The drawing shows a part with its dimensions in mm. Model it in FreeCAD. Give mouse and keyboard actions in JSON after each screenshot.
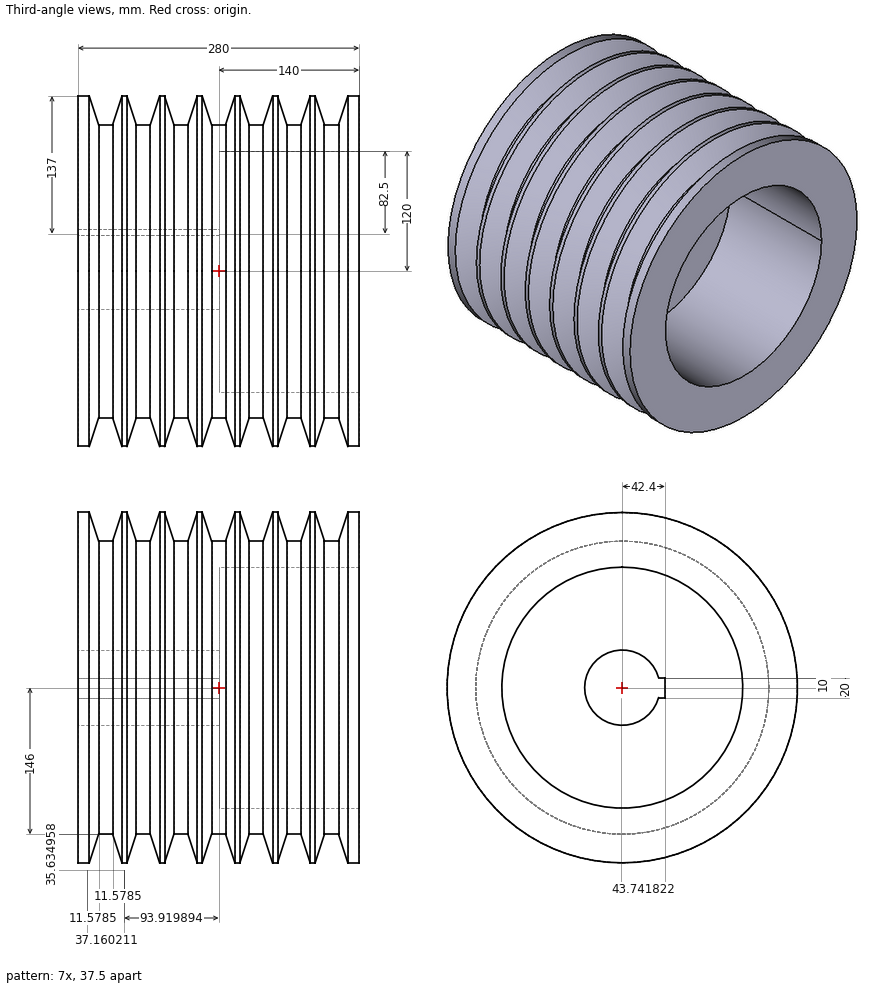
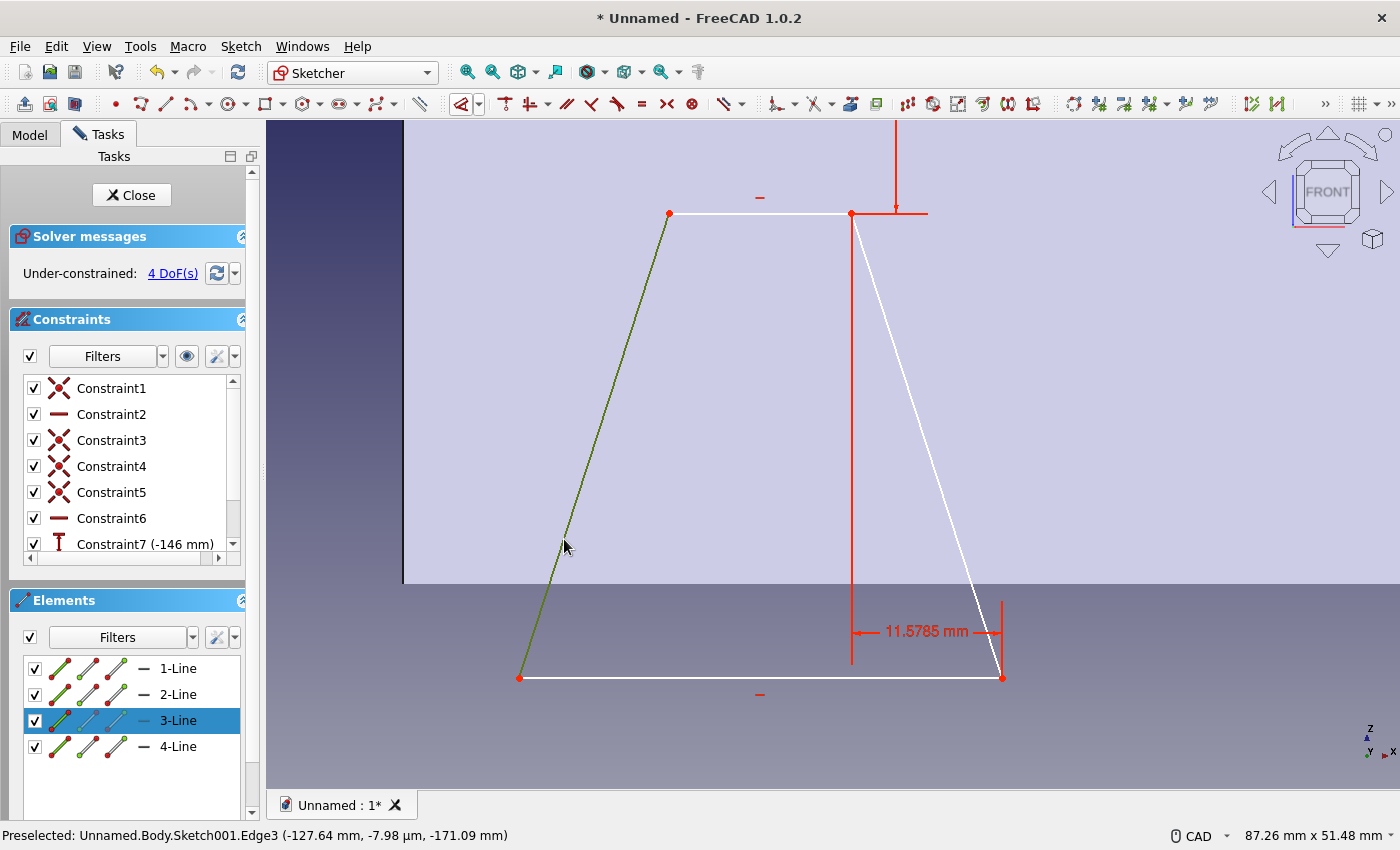
{"action": "left_click", "coordinate": [478, 104]}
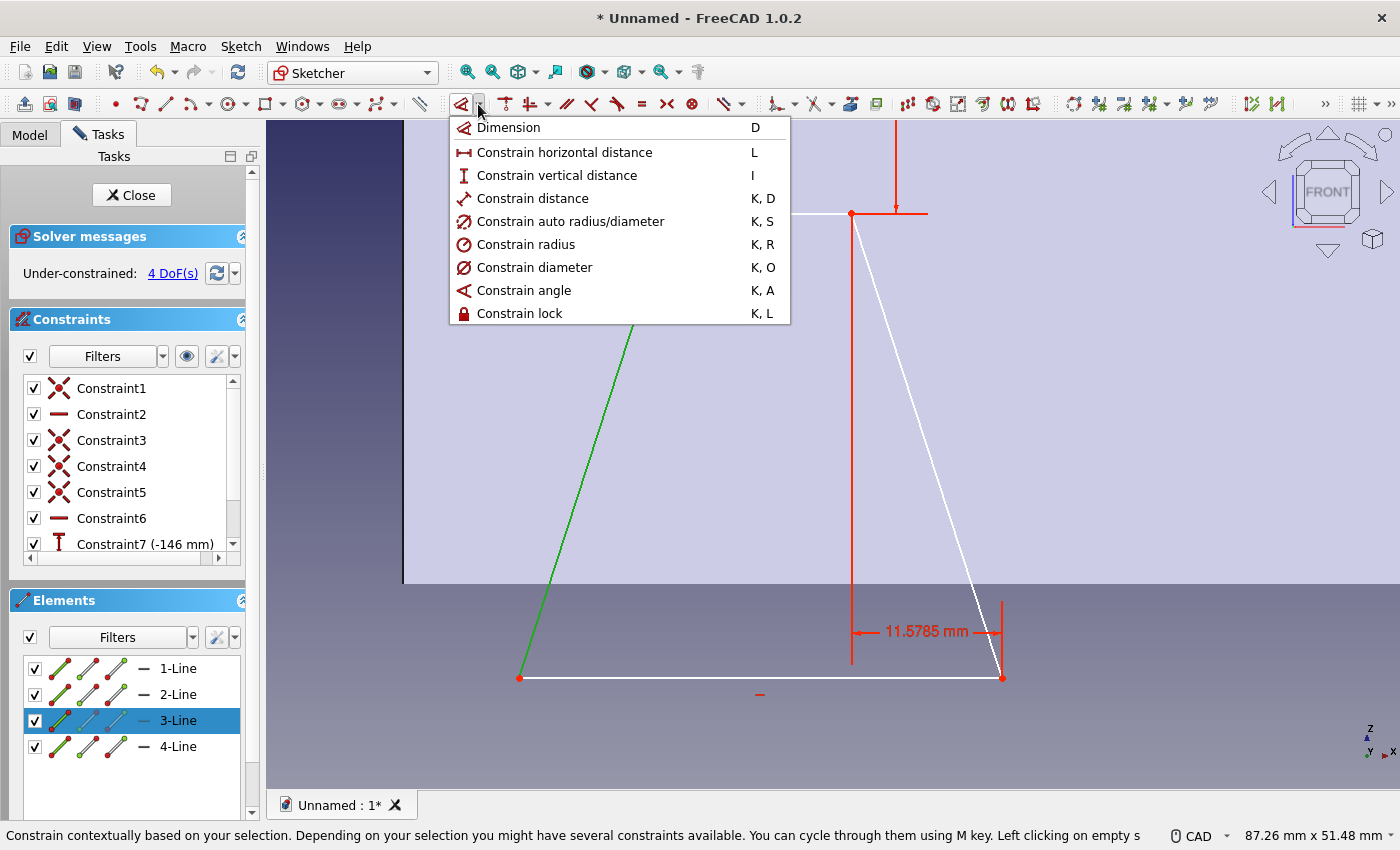
{"action": "left_click", "coordinate": [620, 152]}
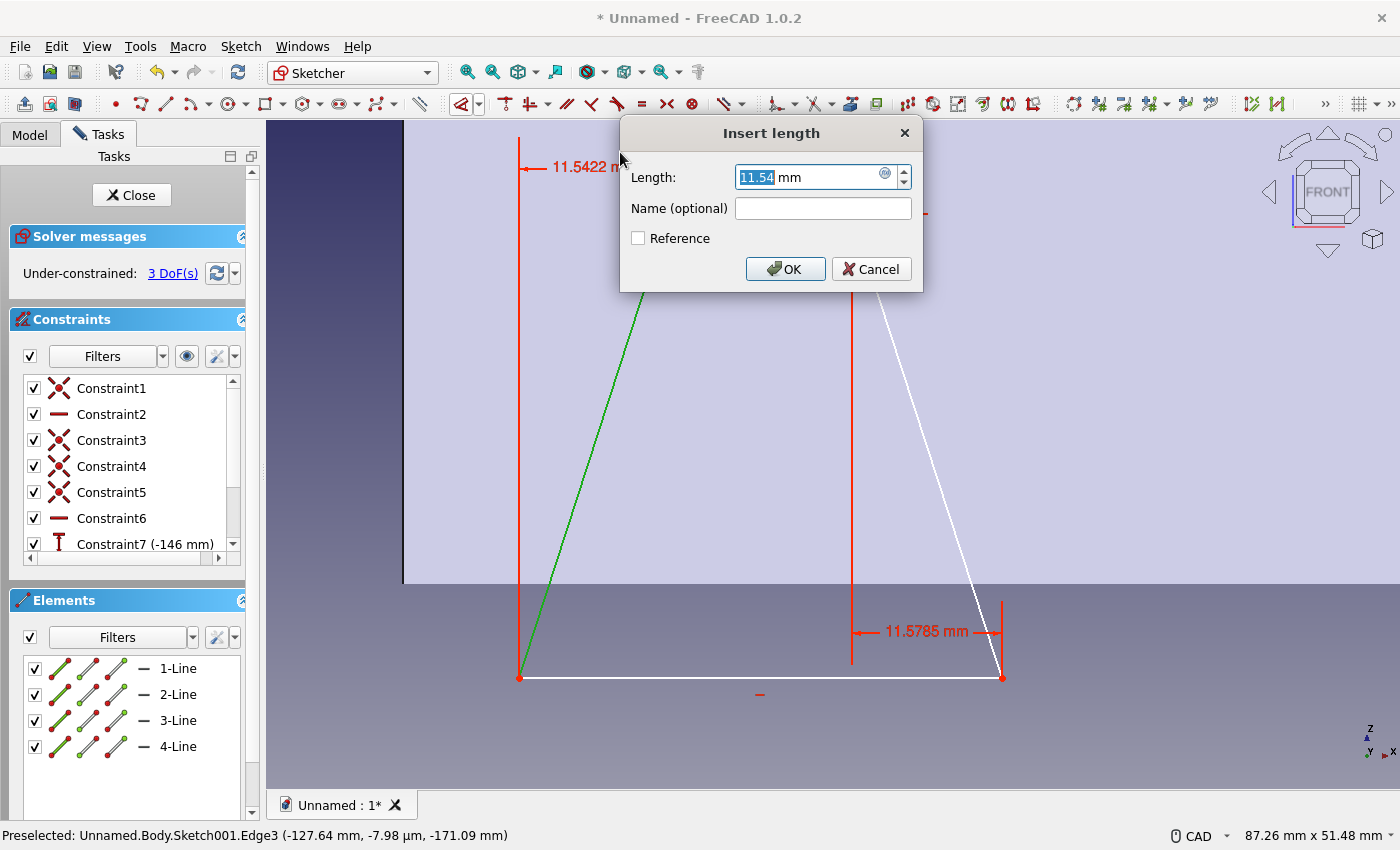
{"action": "type", "text": "11.5785"}
{"action": "key", "text": "Return"}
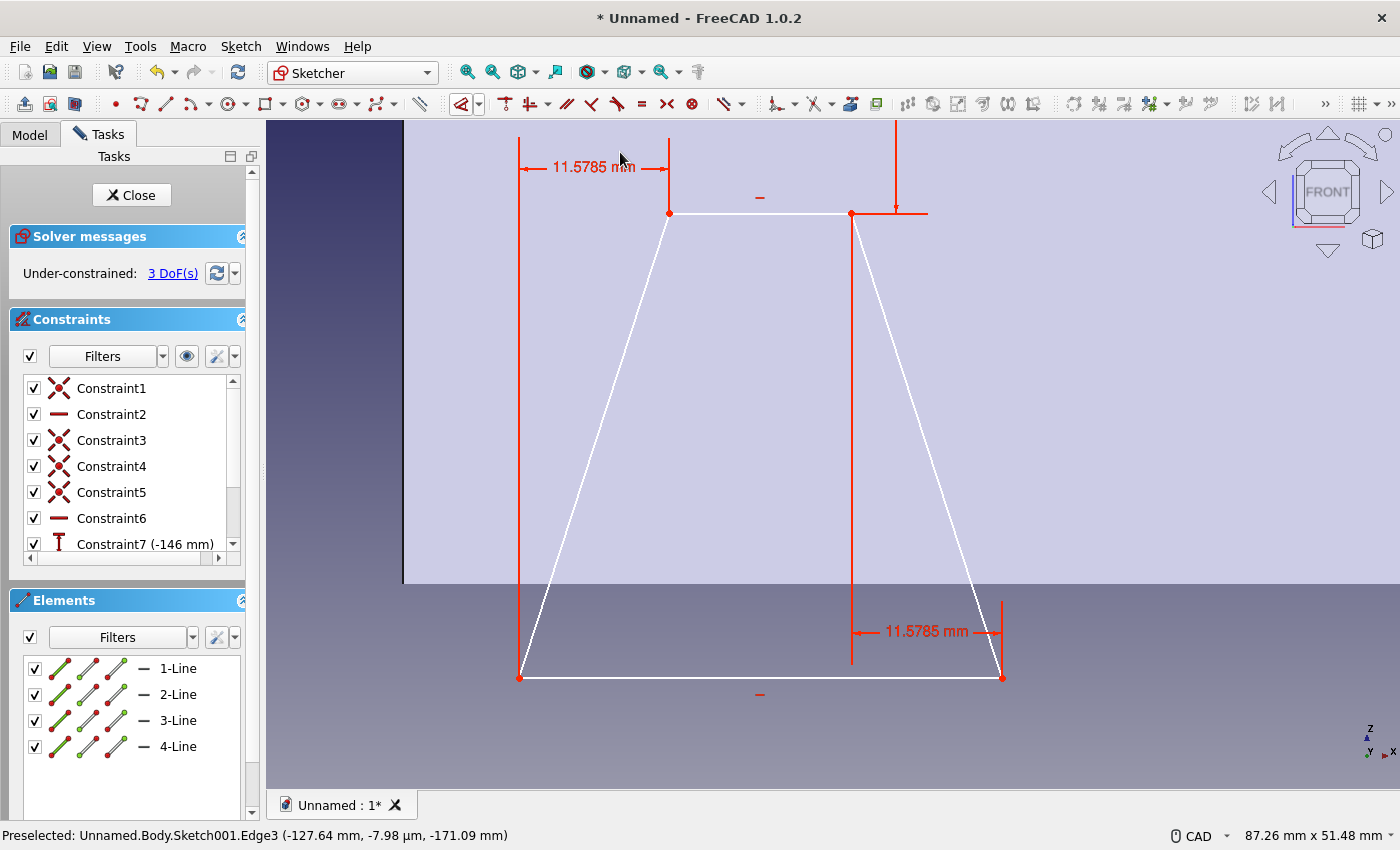
{"action": "left_click", "coordinate": [857, 678]}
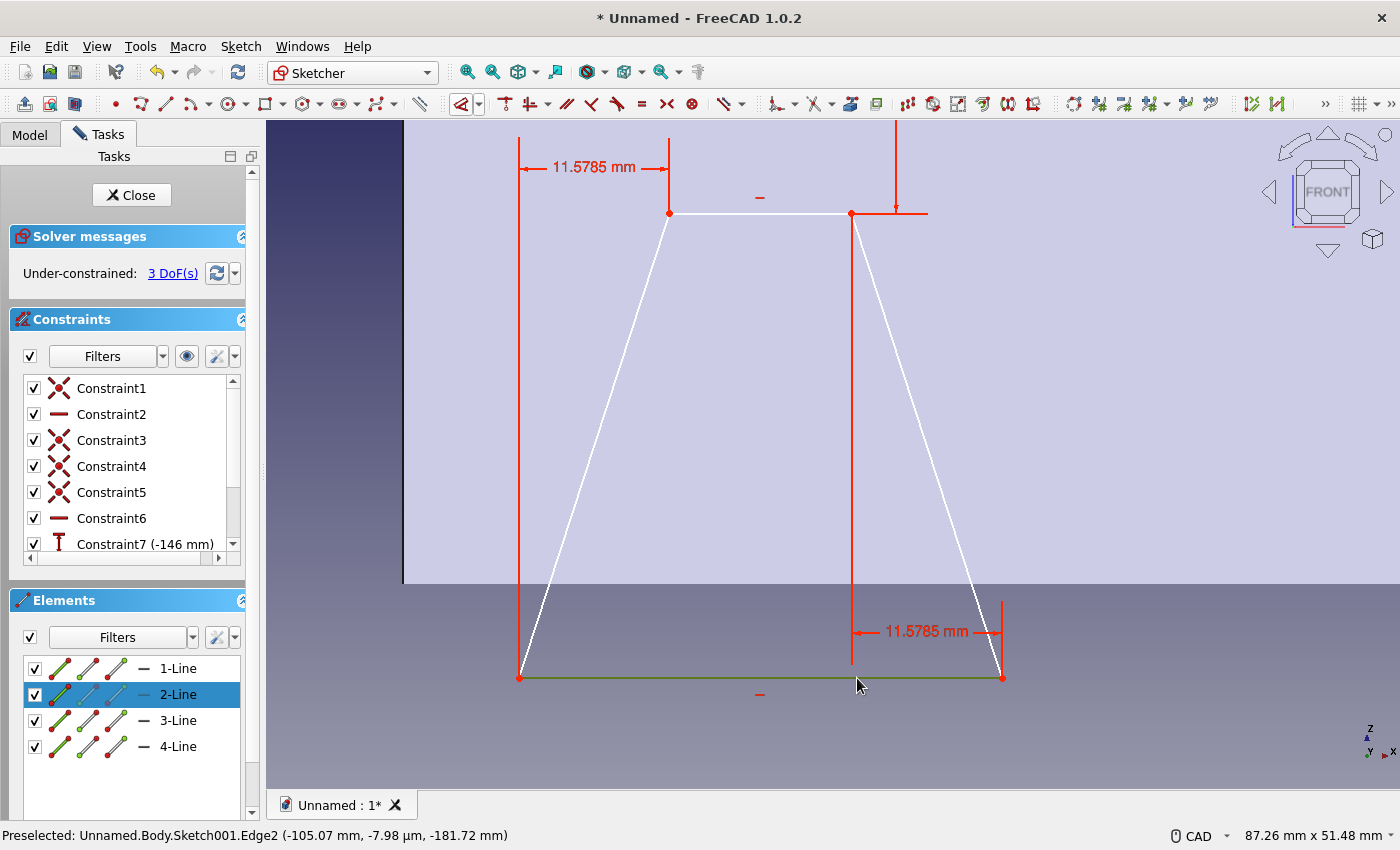
{"action": "left_click", "coordinate": [478, 104]}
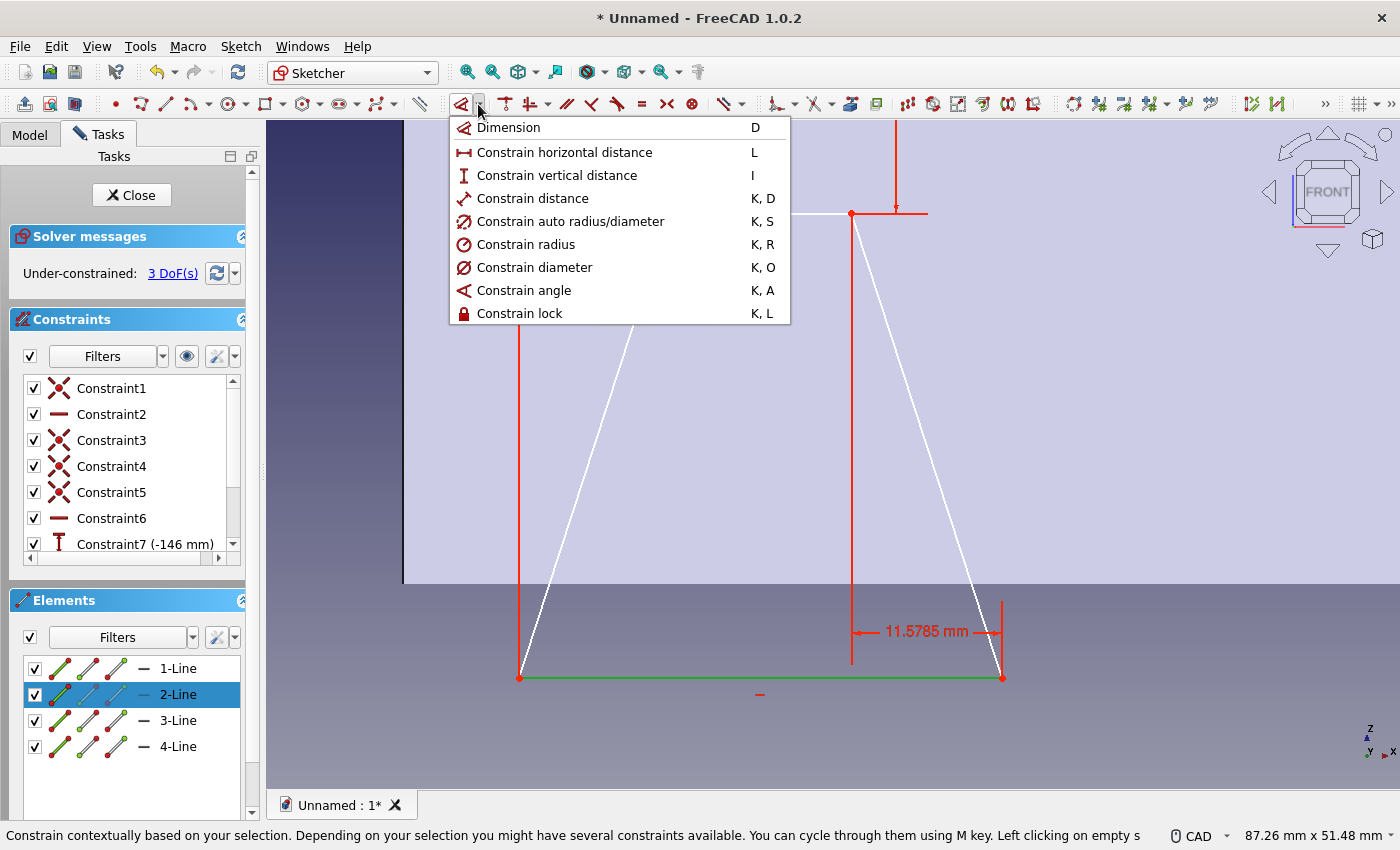
{"action": "left_click", "coordinate": [620, 152]}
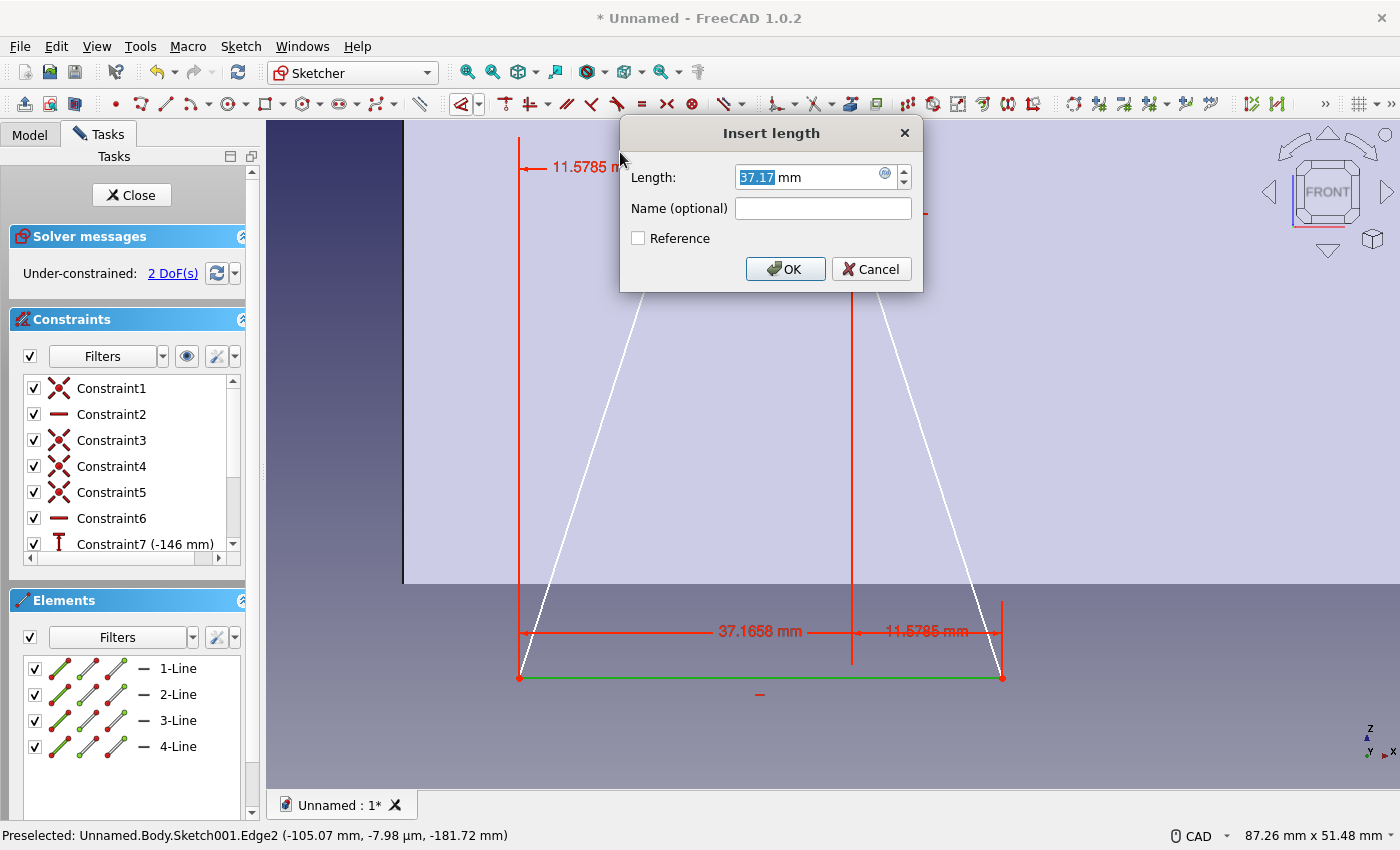
{"action": "type", "text": "37.160211"}
{"action": "key", "text": "Return"}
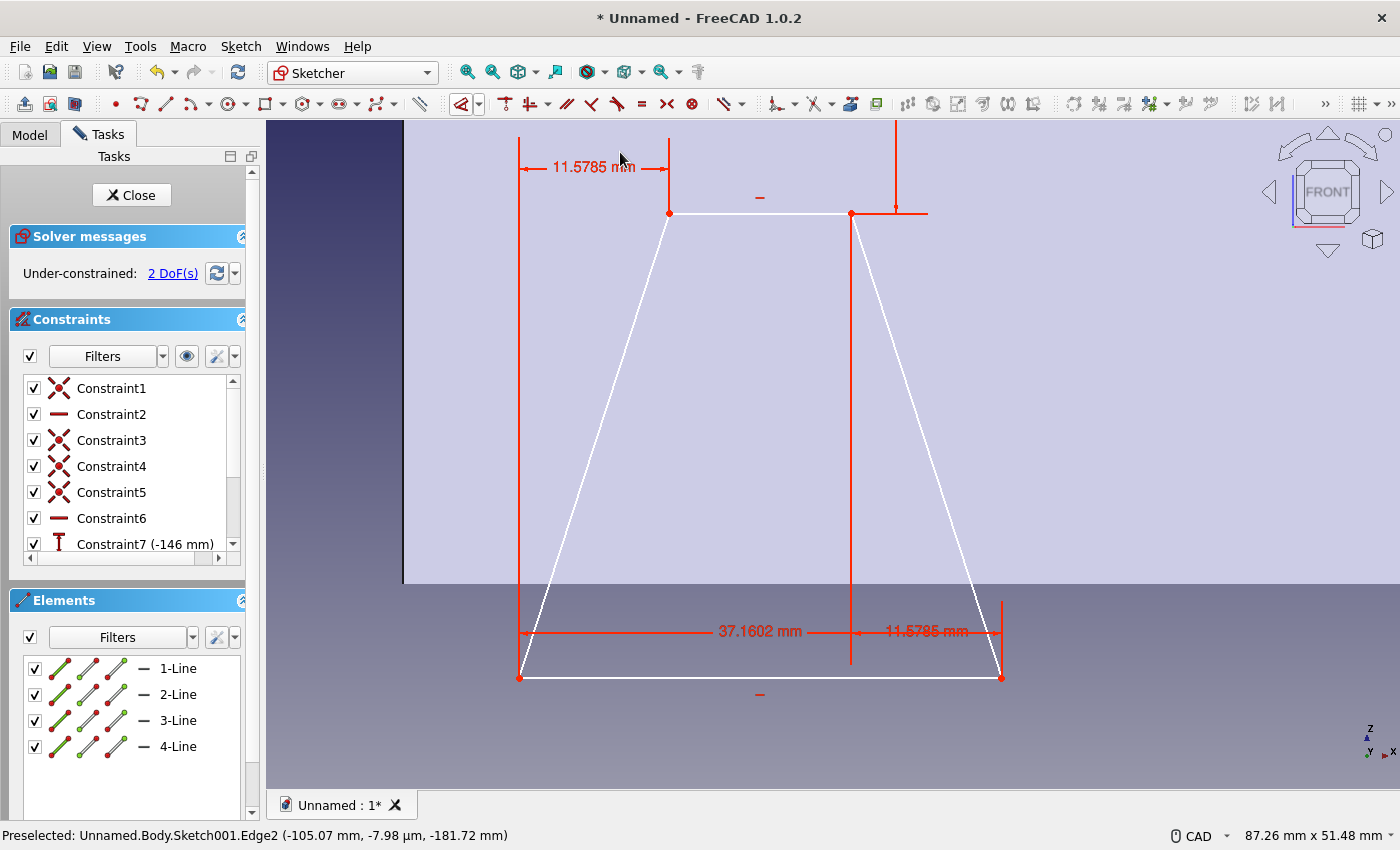
{"action": "left_click", "coordinate": [1002, 678]}